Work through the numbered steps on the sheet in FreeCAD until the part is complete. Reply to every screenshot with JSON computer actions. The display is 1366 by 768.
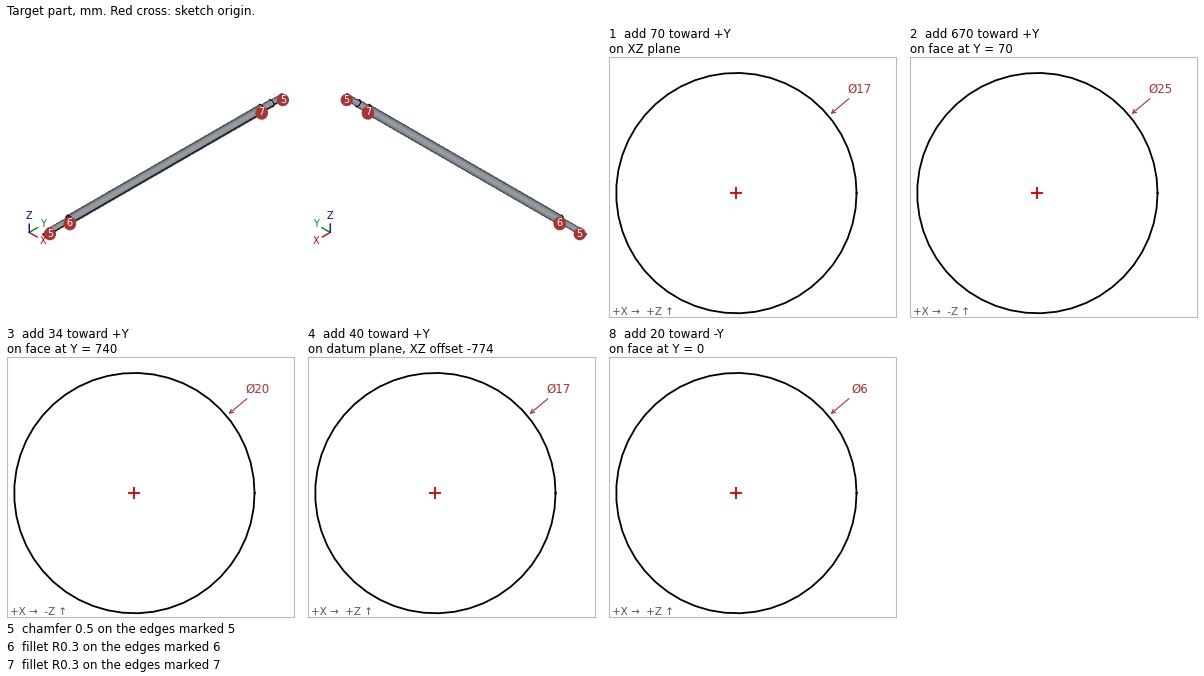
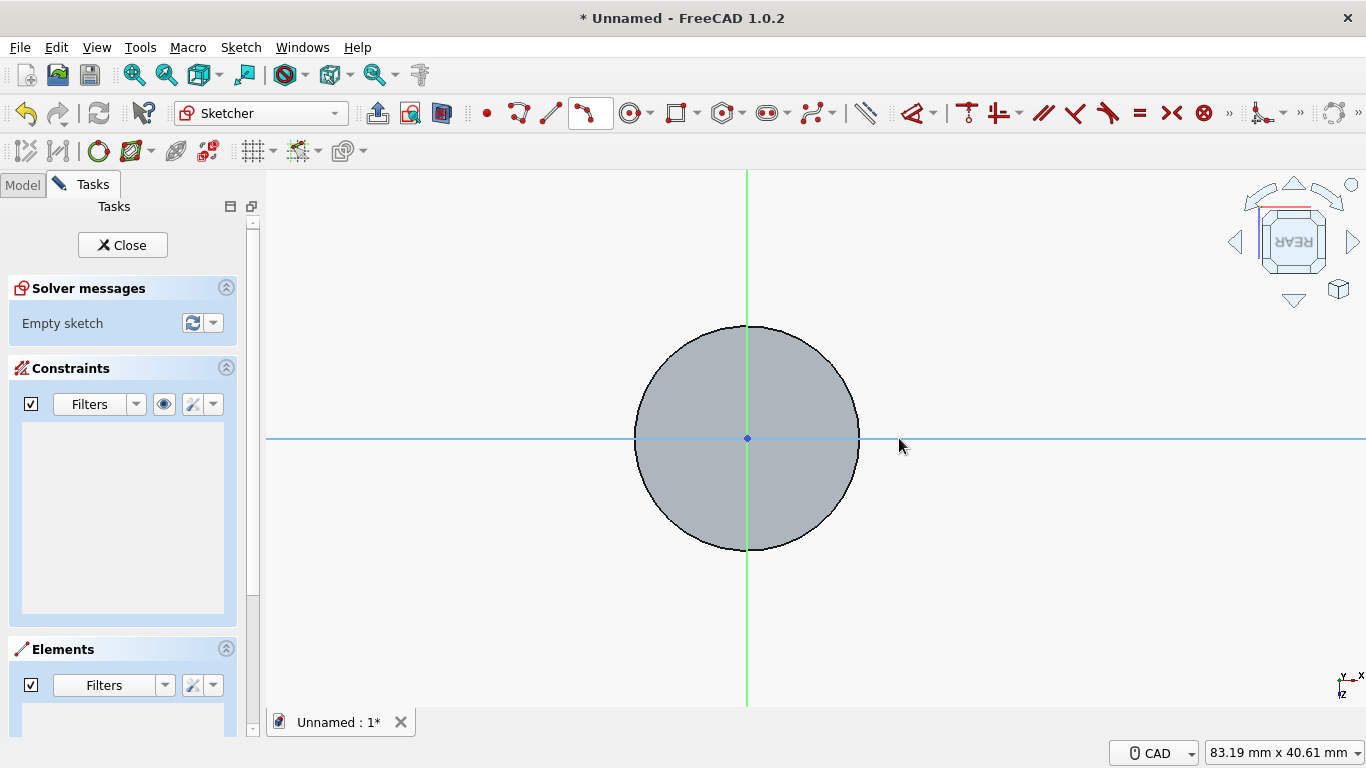
{"action": "key", "text": "g c"}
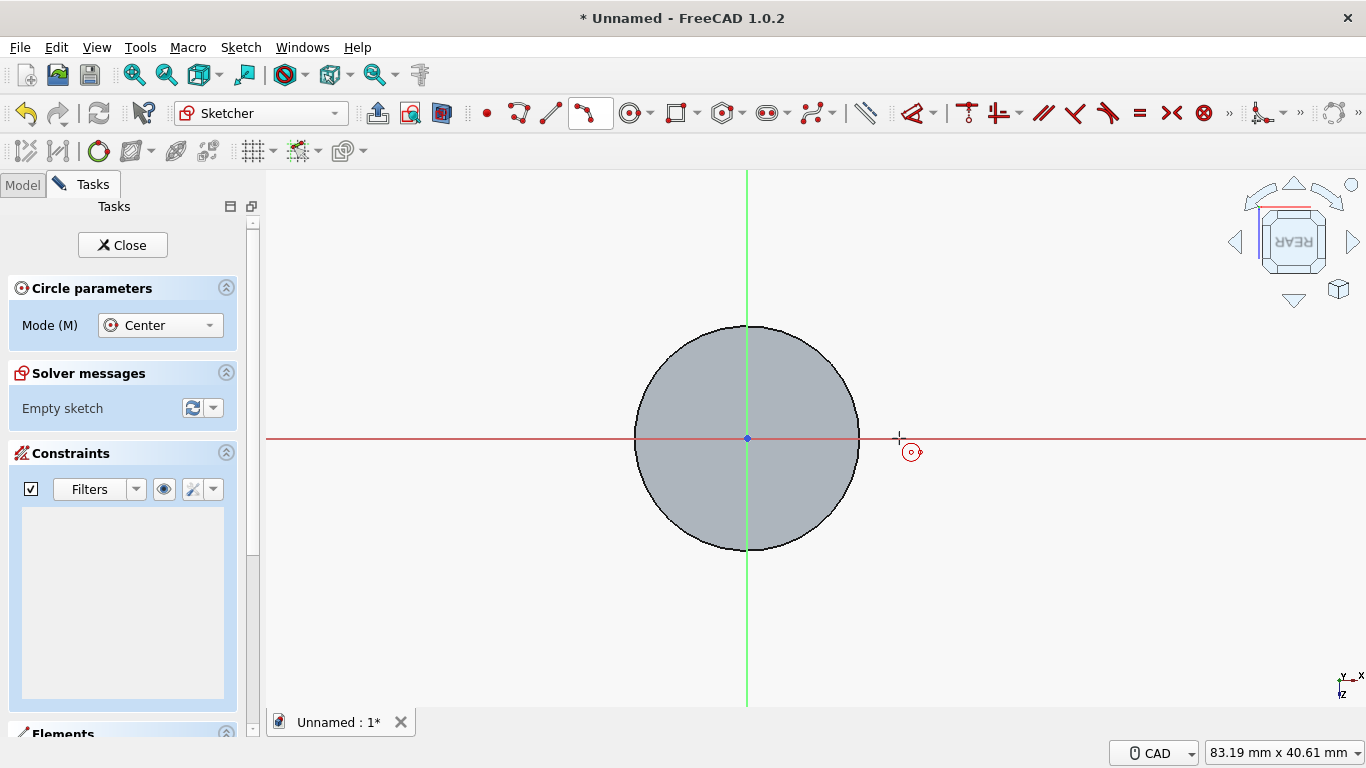
{"action": "left_click", "coordinate": [747, 438]}
{"action": "left_click", "coordinate": [864, 322]}
{"action": "key", "text": "Escape"}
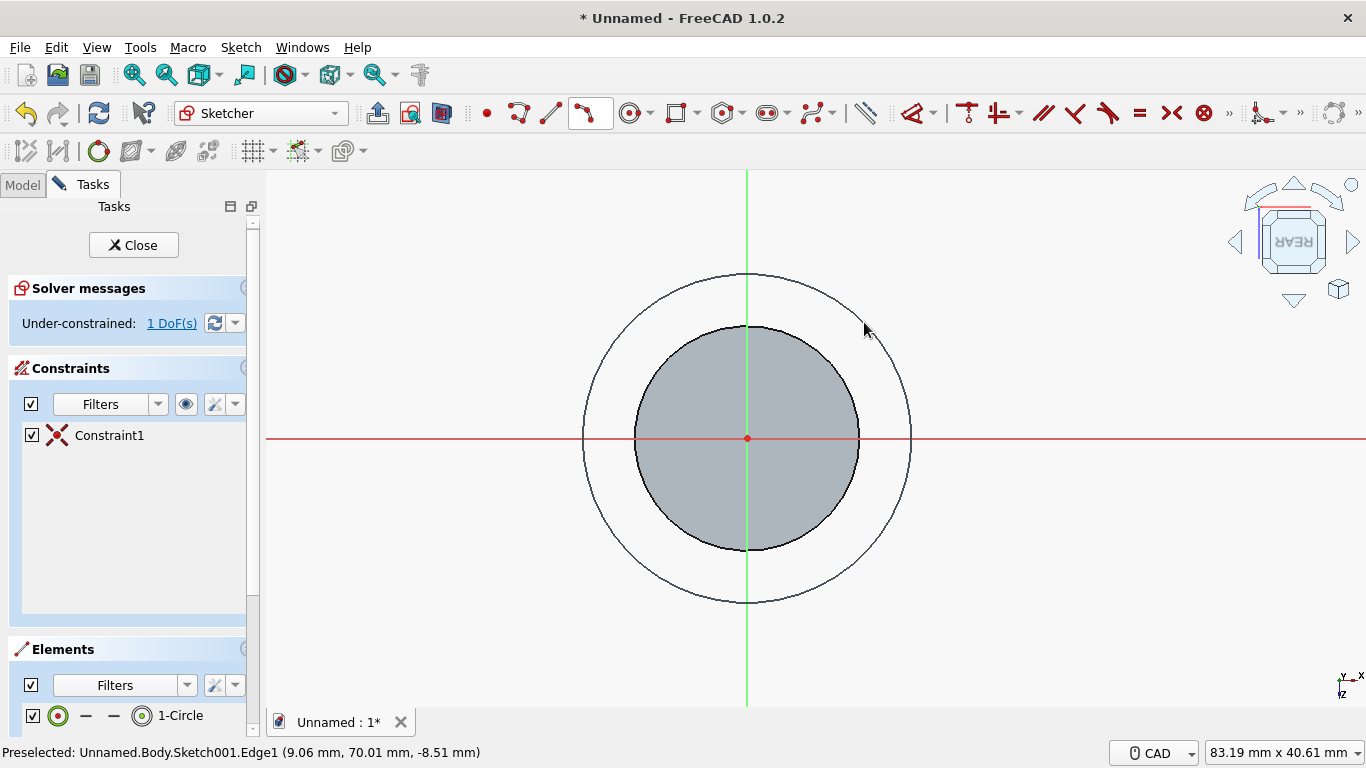
{"action": "left_click", "coordinate": [912, 114]}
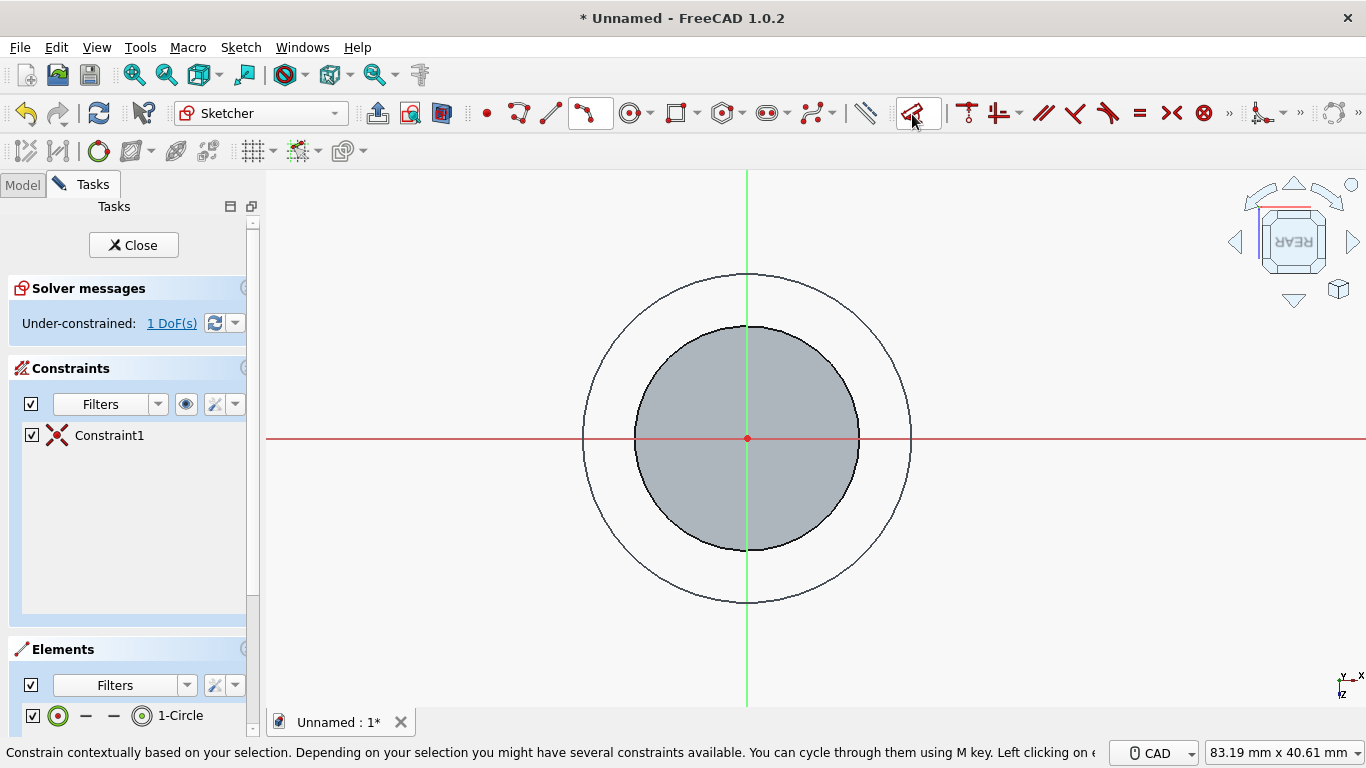
{"action": "left_click", "coordinate": [863, 322]}
{"action": "left_click", "coordinate": [886, 299]}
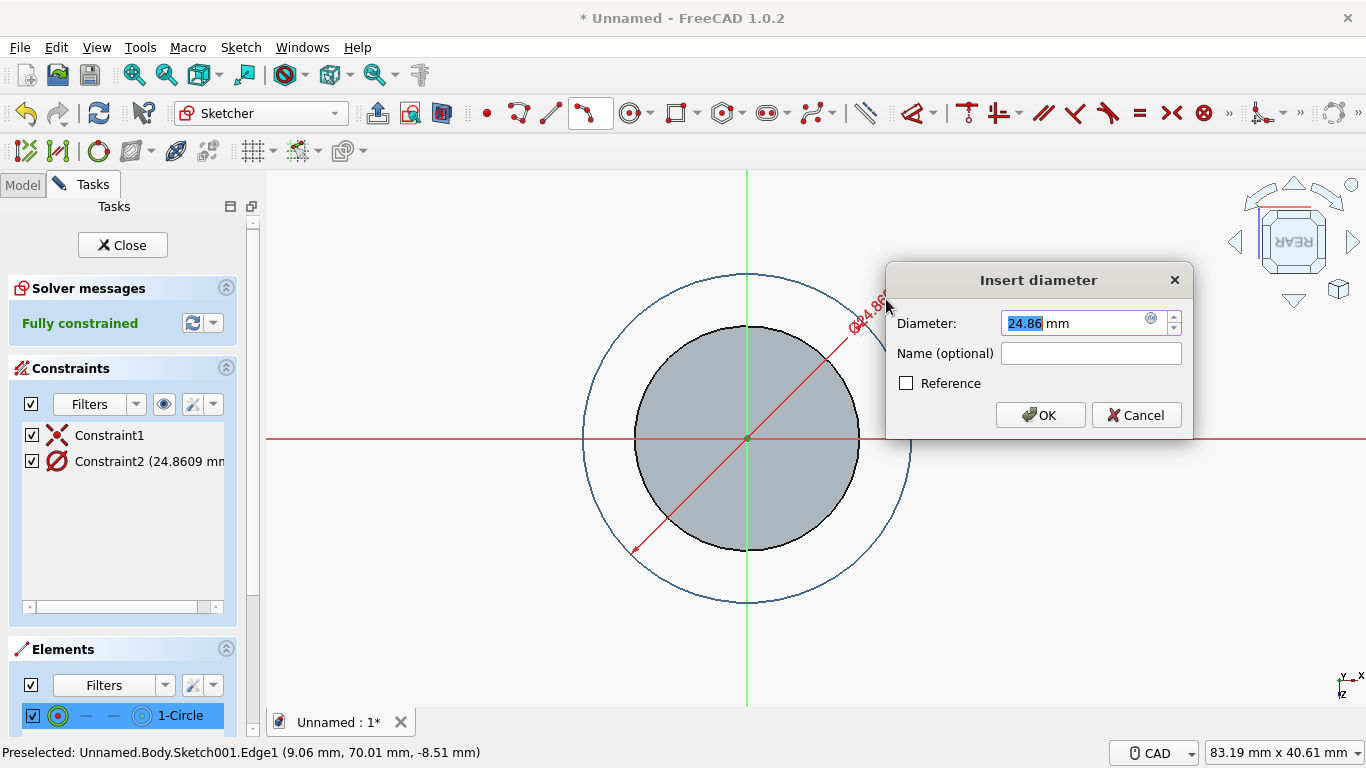
{"action": "type", "text": "25"}
{"action": "key", "text": "Return"}
{"action": "key", "text": "Escape"}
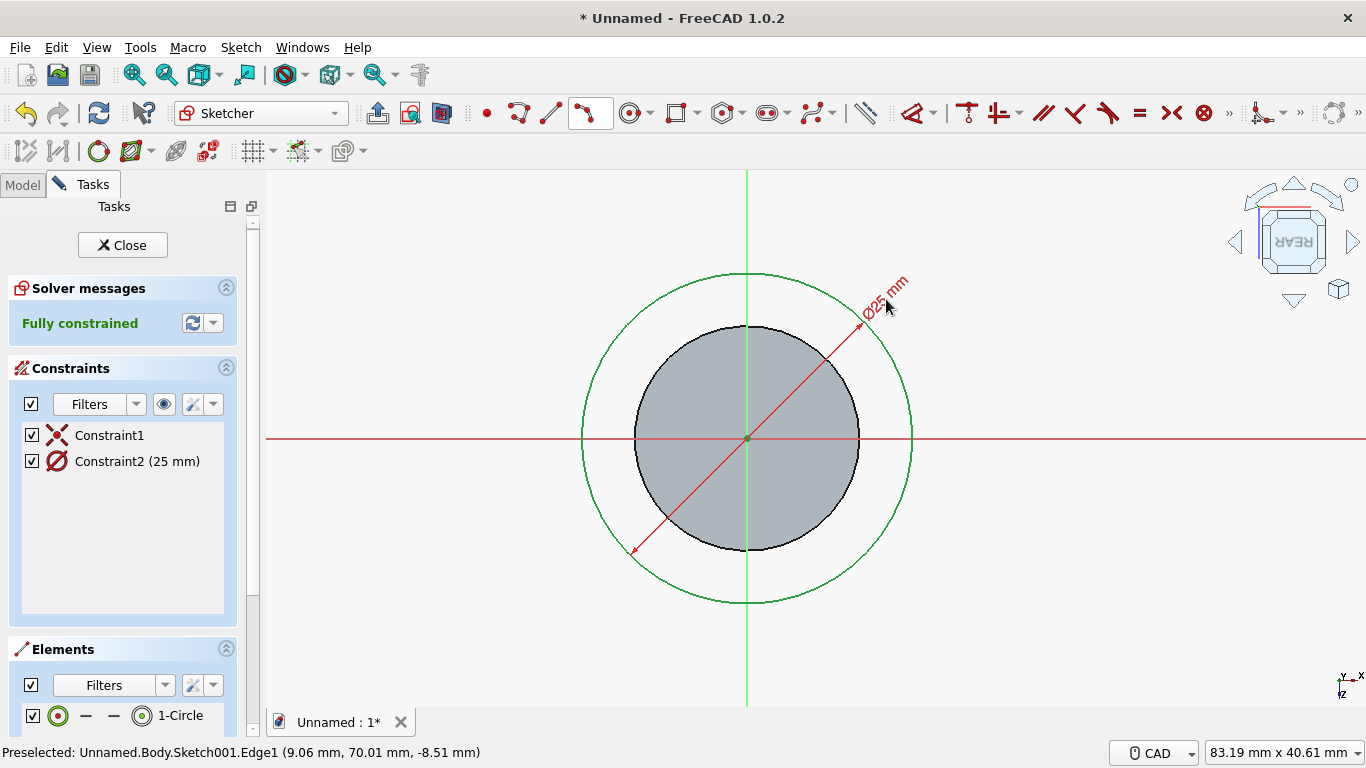
{"action": "left_click", "coordinate": [123, 245]}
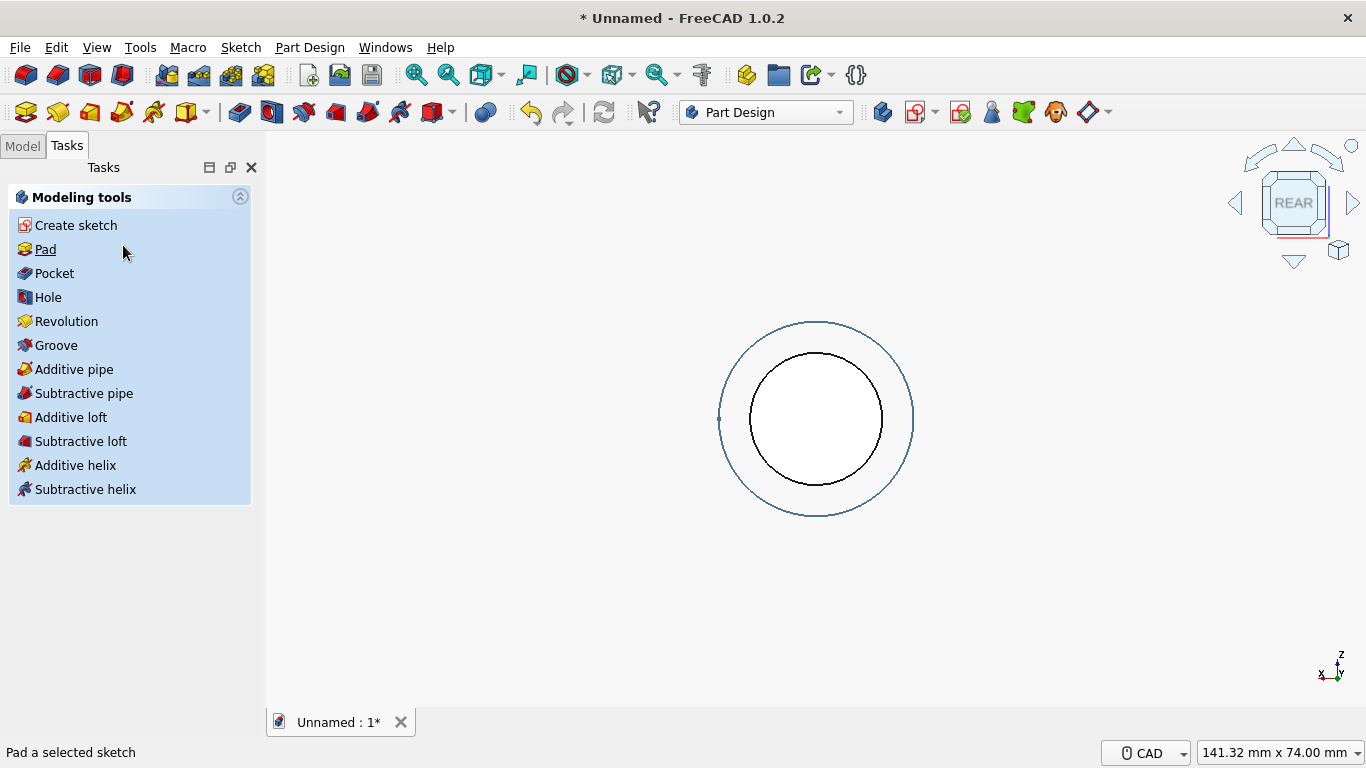
{"action": "left_click", "coordinate": [26, 112]}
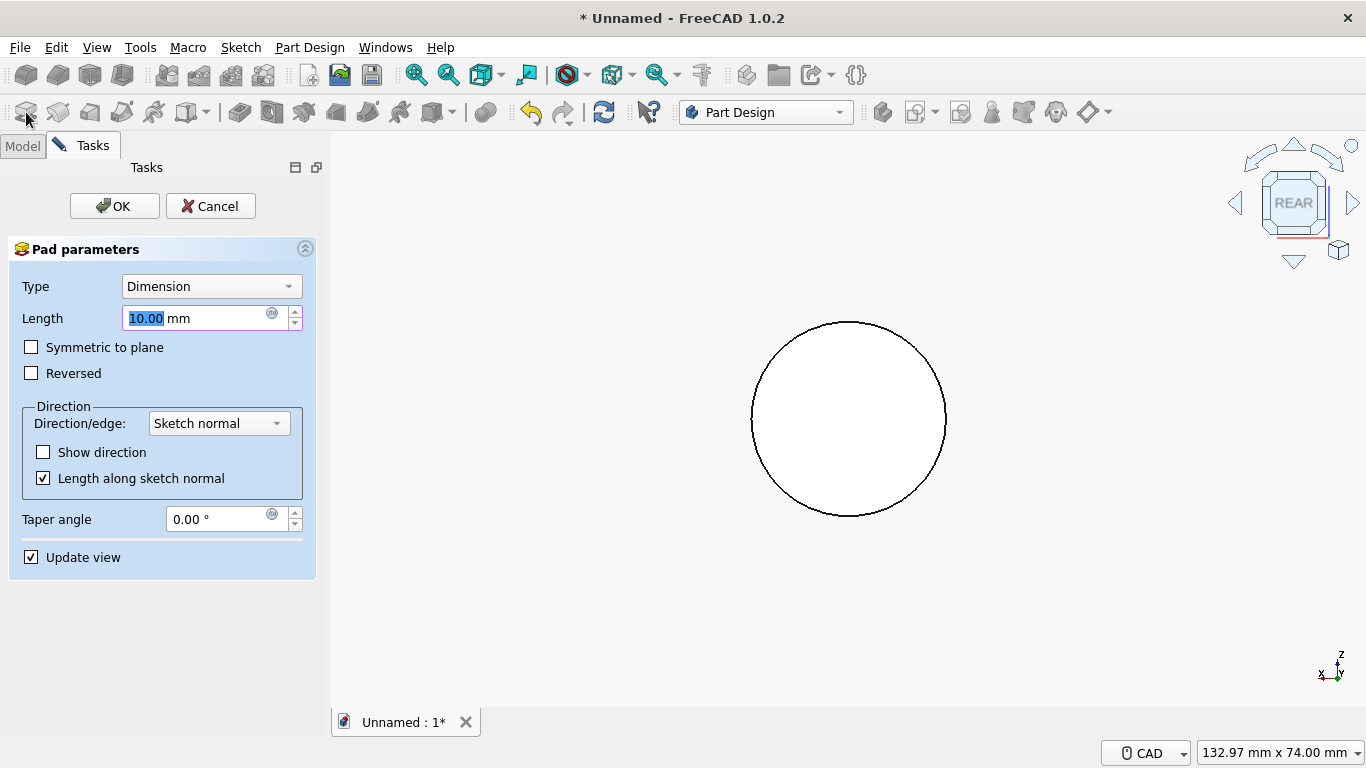
{"action": "type", "text": "670"}
{"action": "key", "text": "Tab"}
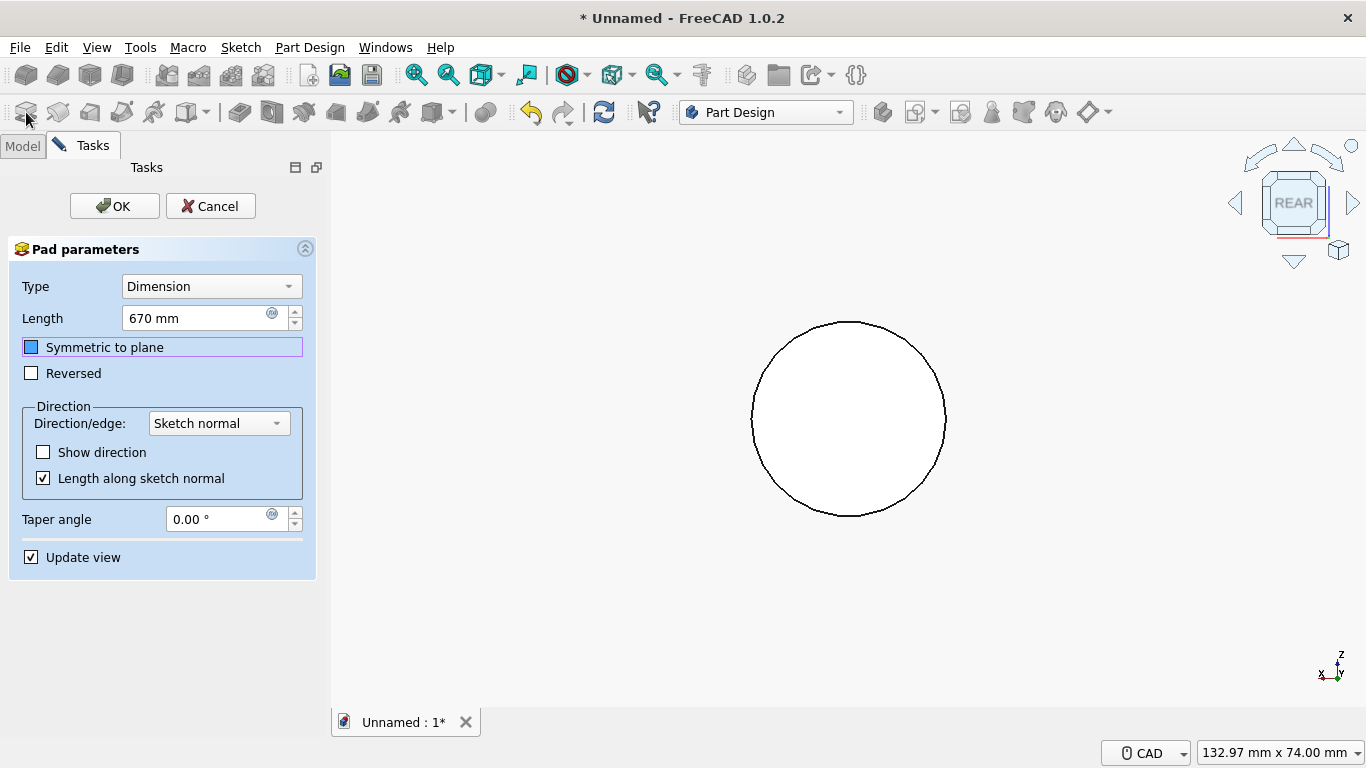
{"action": "left_click", "coordinate": [115, 206]}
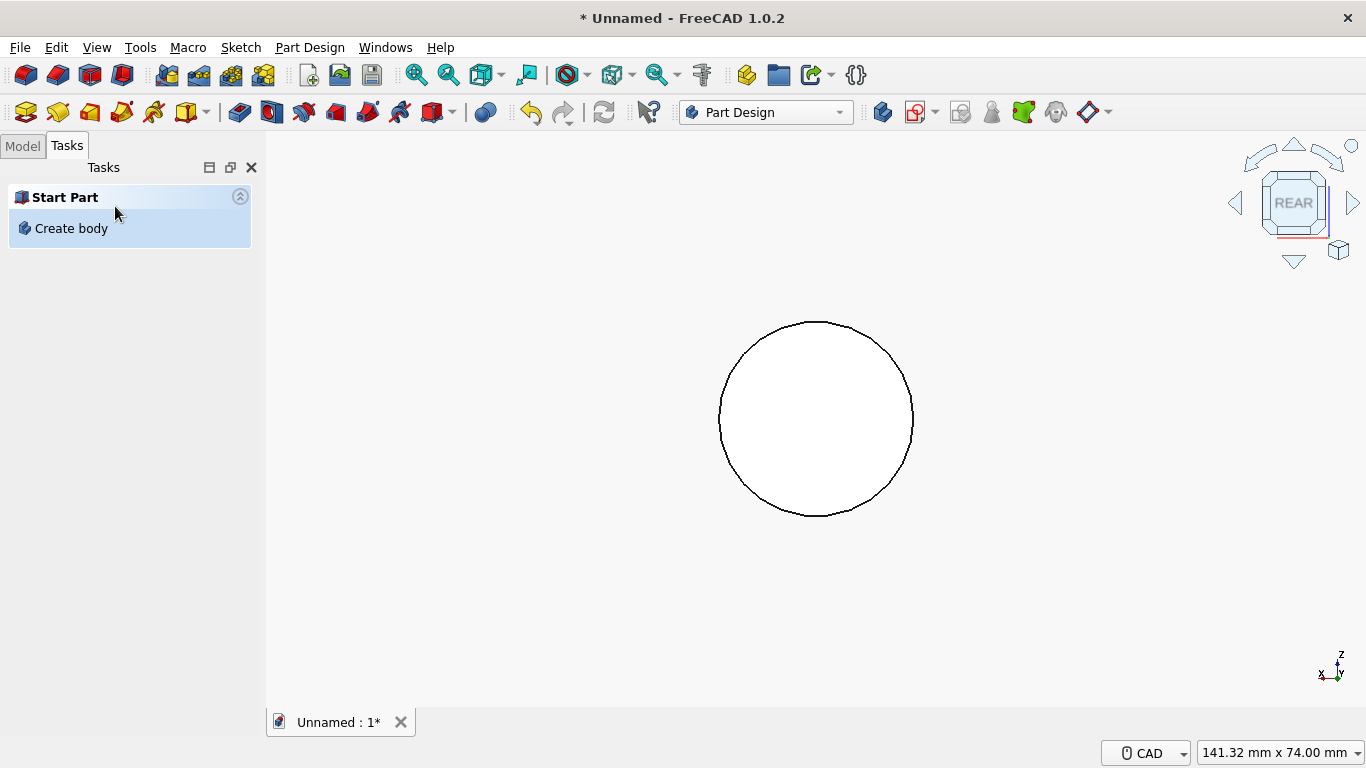
{"action": "left_click", "coordinate": [418, 76]}